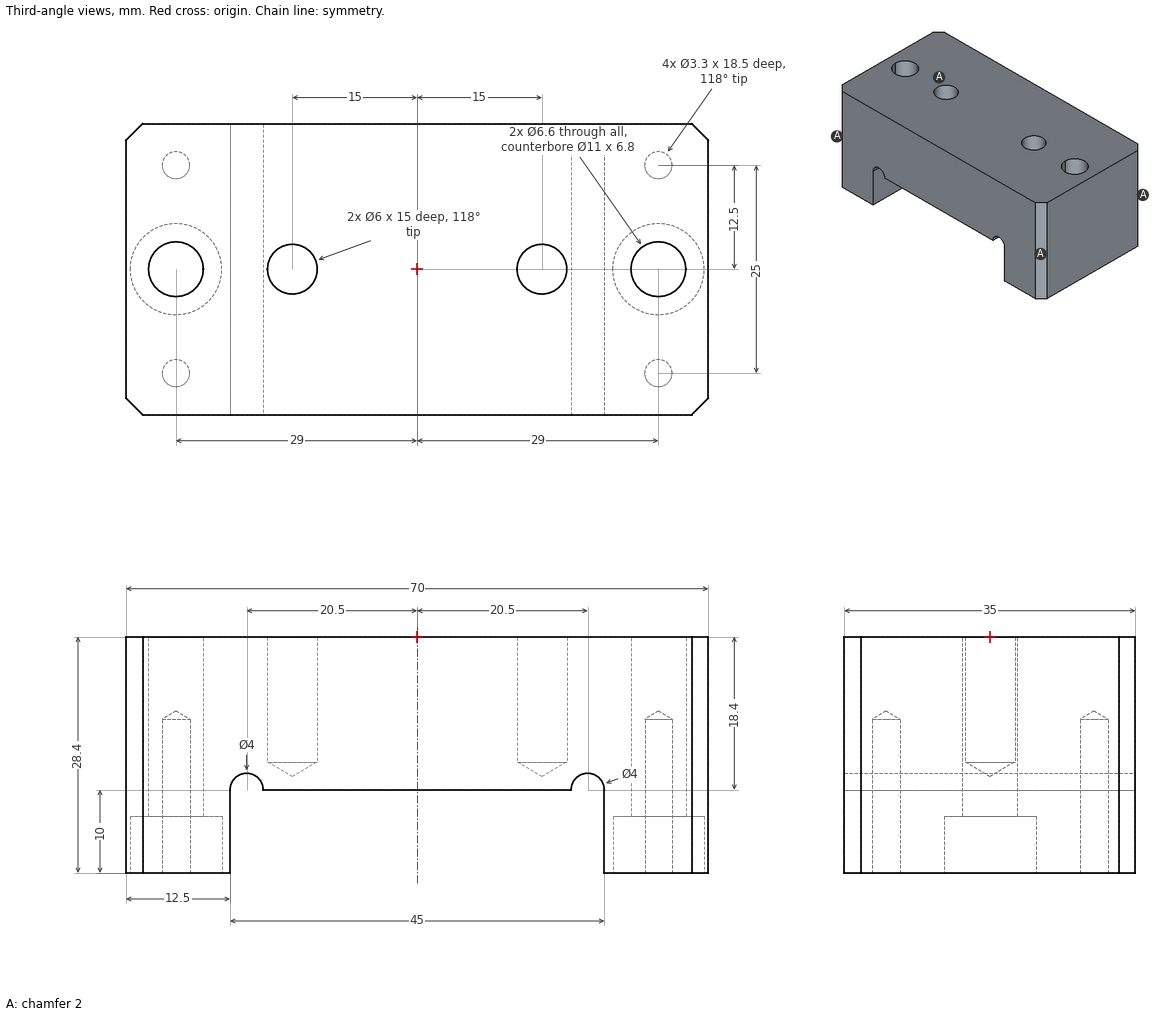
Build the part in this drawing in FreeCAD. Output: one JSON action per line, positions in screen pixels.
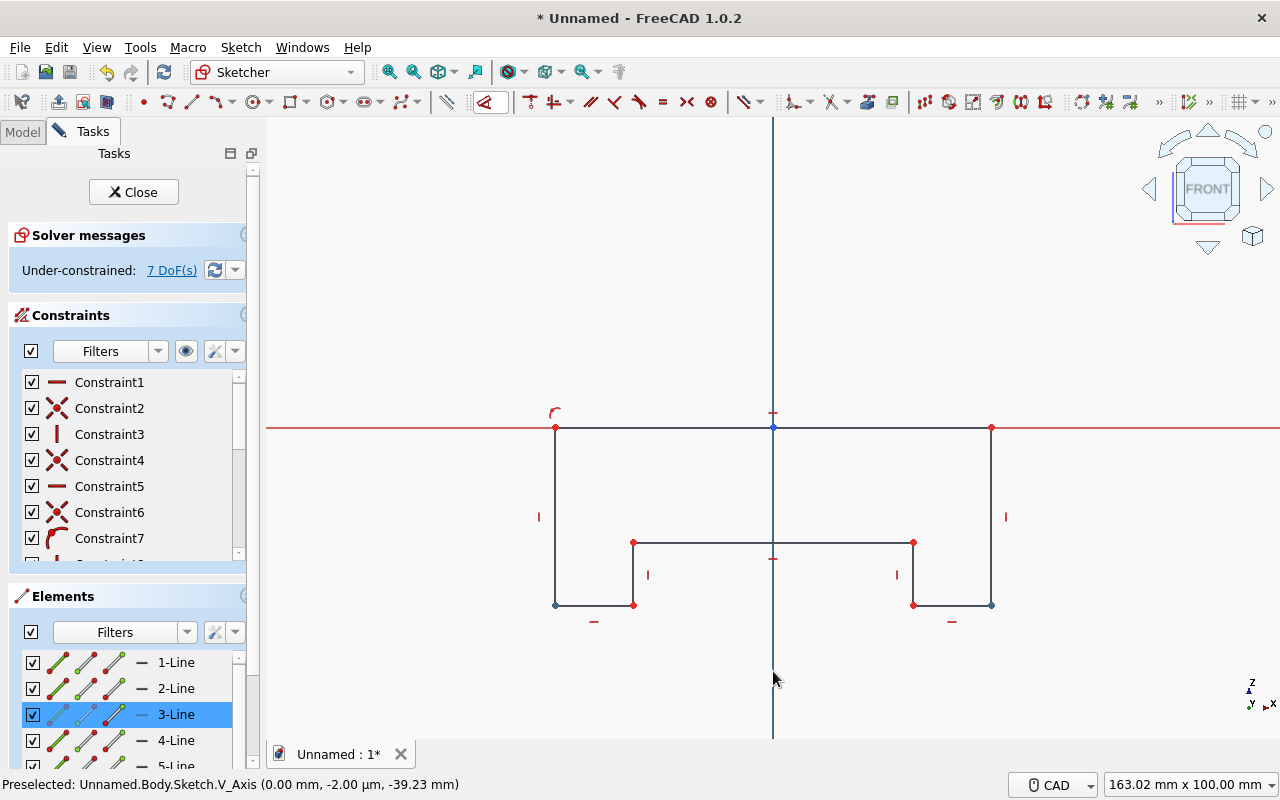
{"action": "key", "text": "s"}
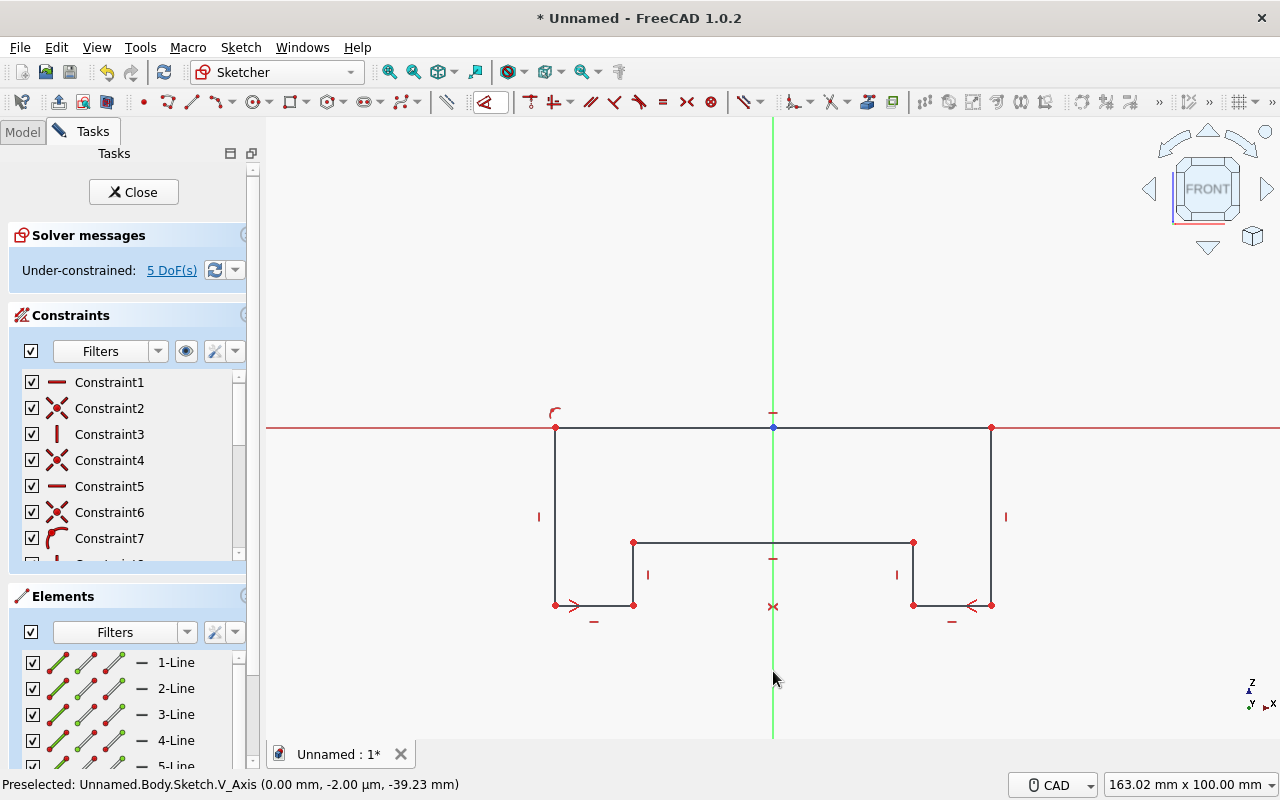
{"action": "key", "text": "d"}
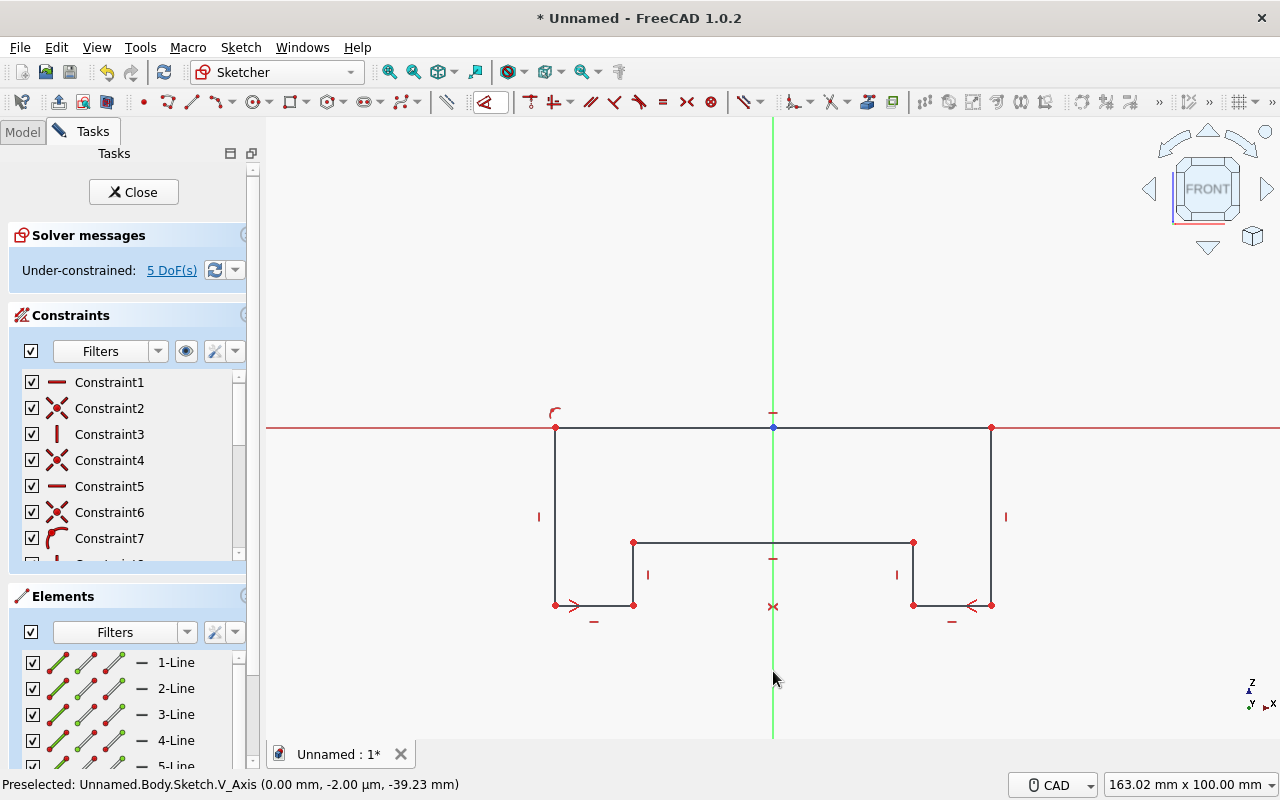
{"action": "left_click", "coordinate": [829, 543]}
{"action": "left_click", "coordinate": [709, 577]}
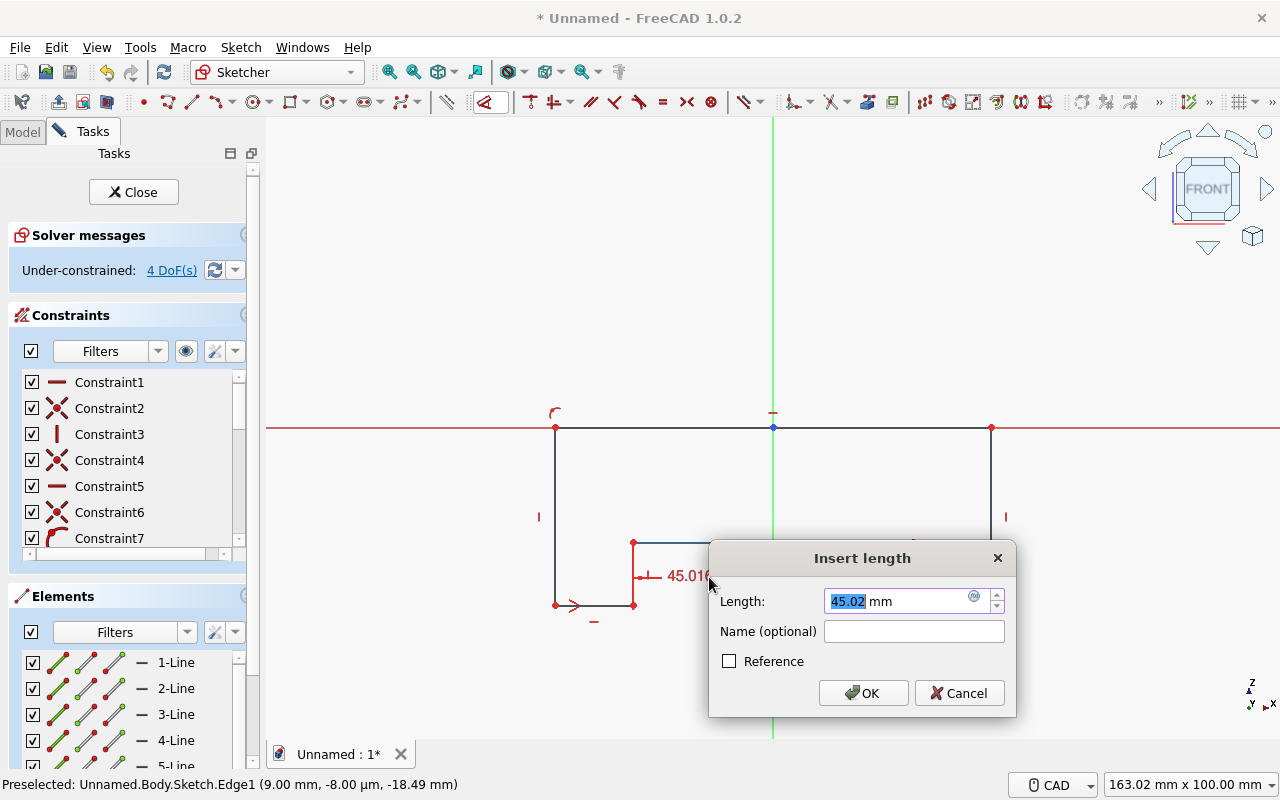
{"action": "type", "text": "45"}
{"action": "key", "text": "Return"}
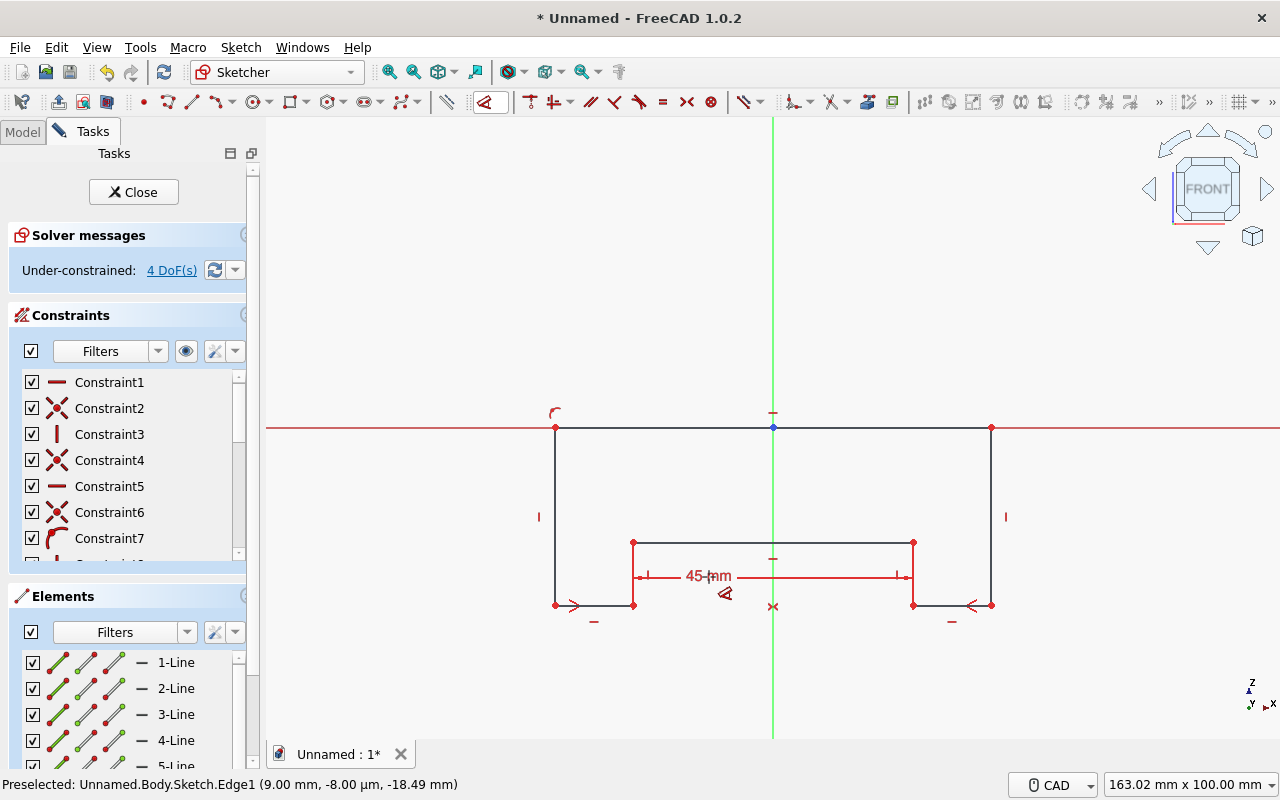
{"action": "left_click", "coordinate": [633, 562]}
{"action": "left_click", "coordinate": [599, 575]}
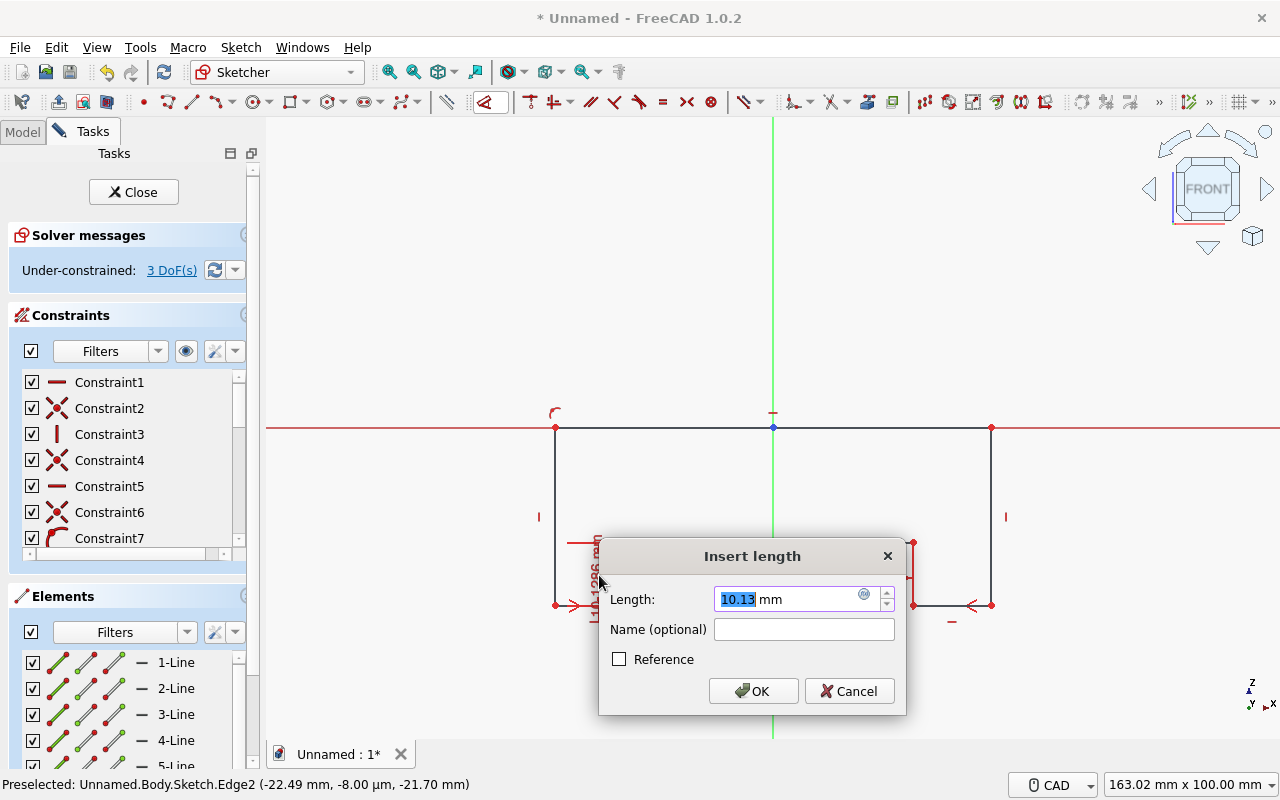
{"action": "type", "text": "10"}
{"action": "key", "text": "Return"}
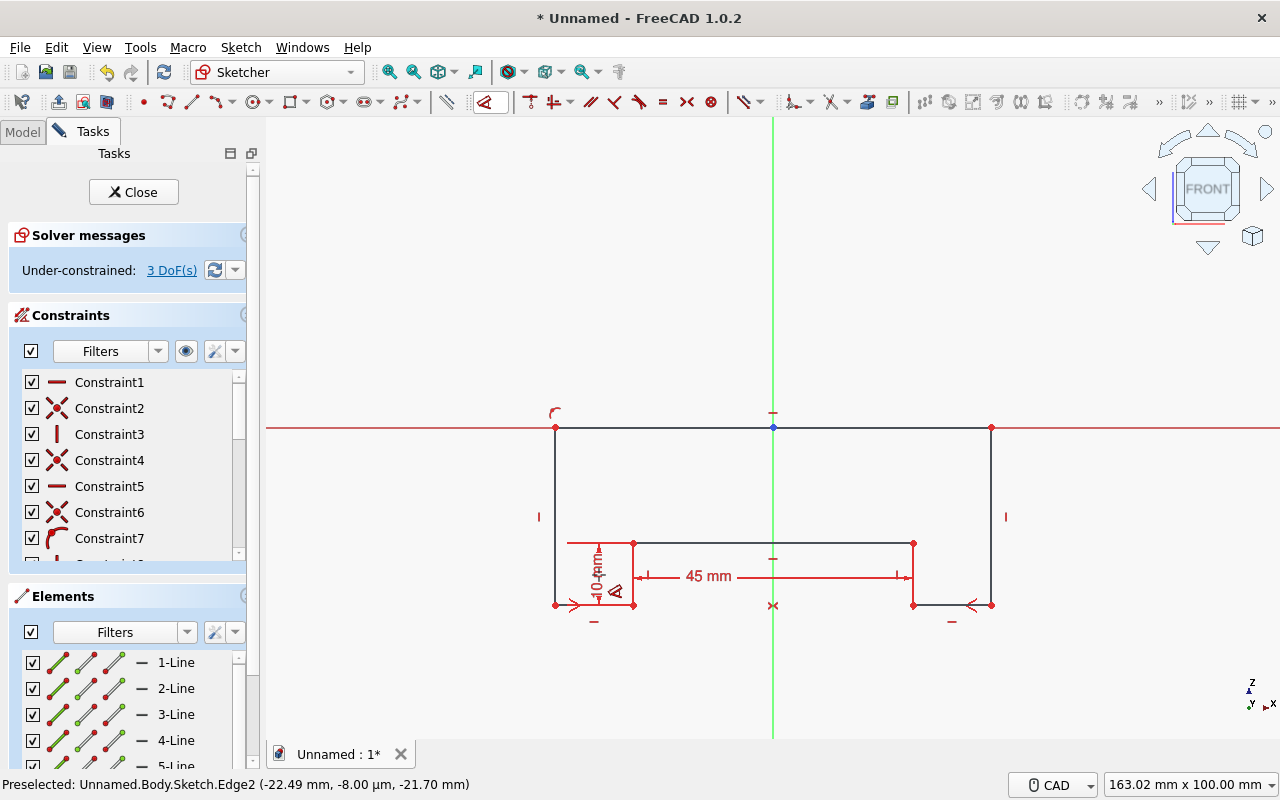
{"action": "left_click", "coordinate": [686, 428]}
{"action": "left_click", "coordinate": [673, 394]}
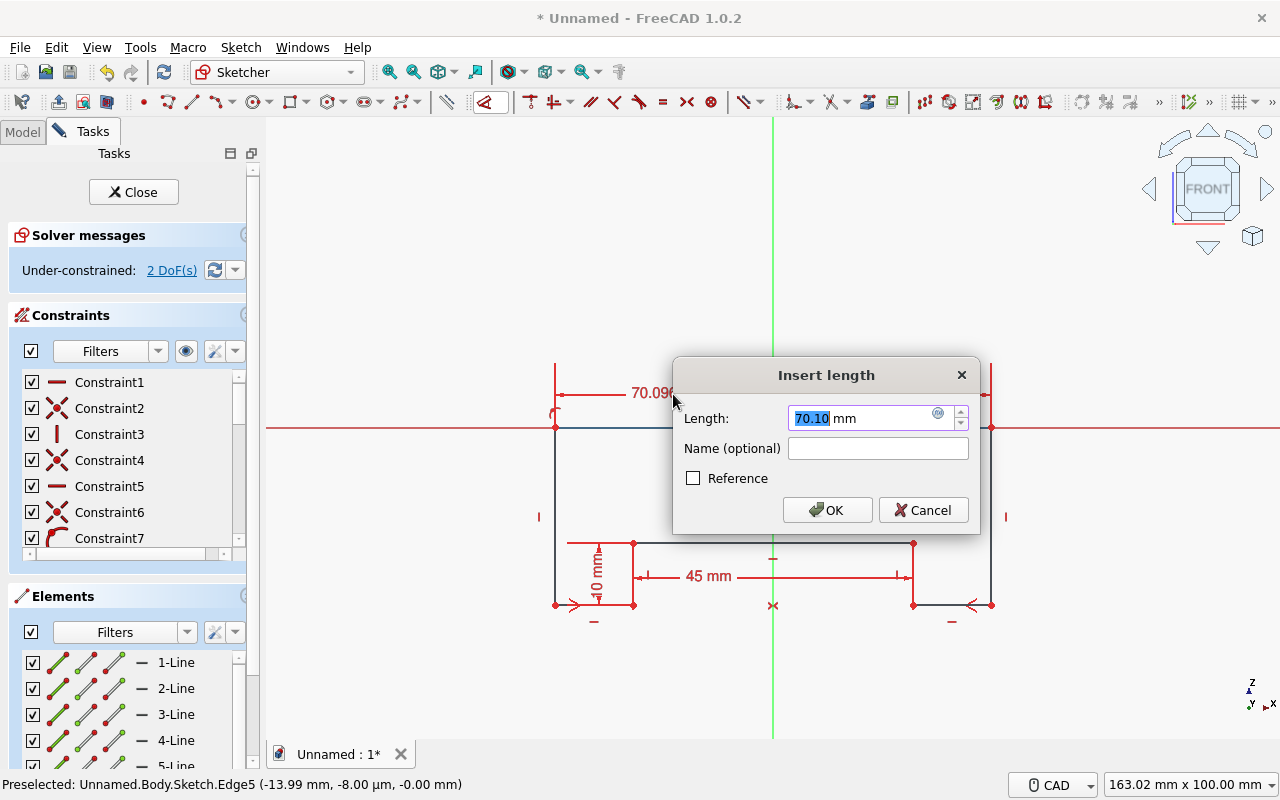
{"action": "type", "text": "70"}
{"action": "key", "text": "Return"}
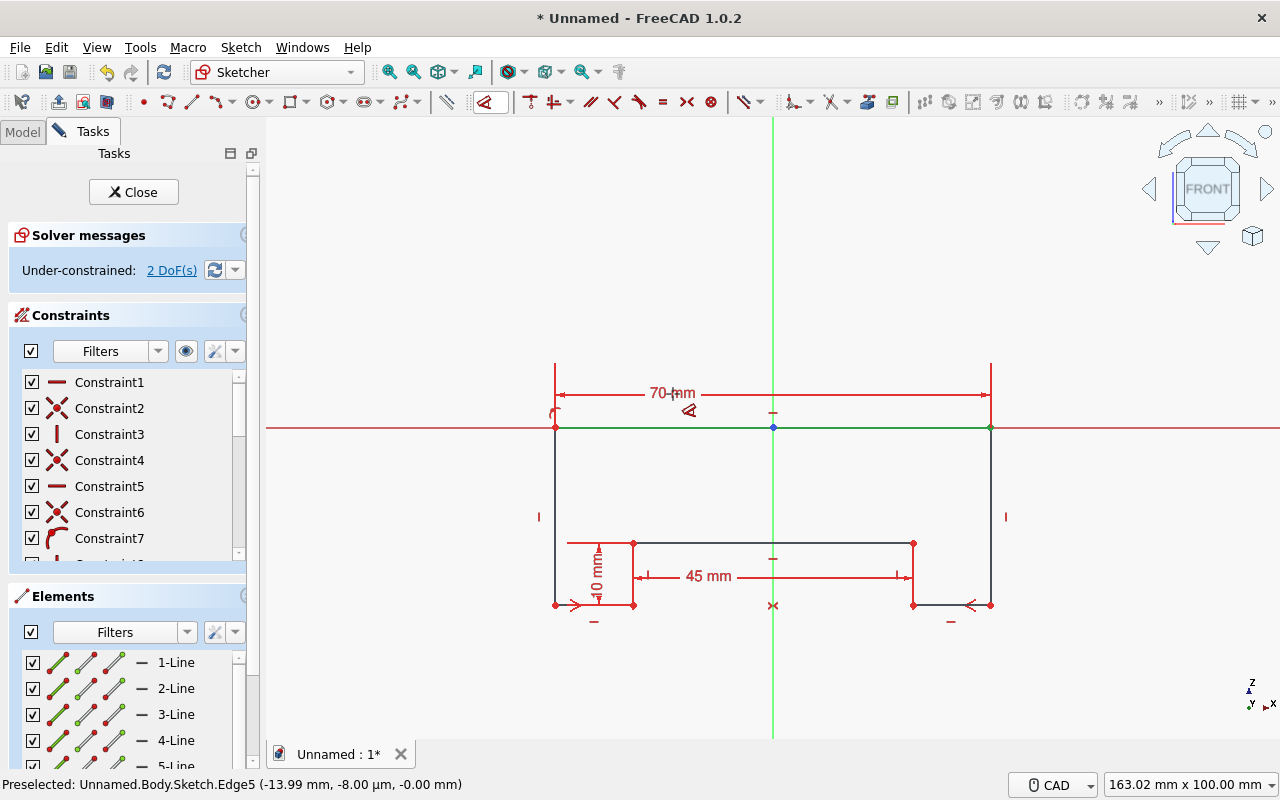
{"action": "left_click", "coordinate": [610, 605]}
{"action": "left_click", "coordinate": [594, 639]}